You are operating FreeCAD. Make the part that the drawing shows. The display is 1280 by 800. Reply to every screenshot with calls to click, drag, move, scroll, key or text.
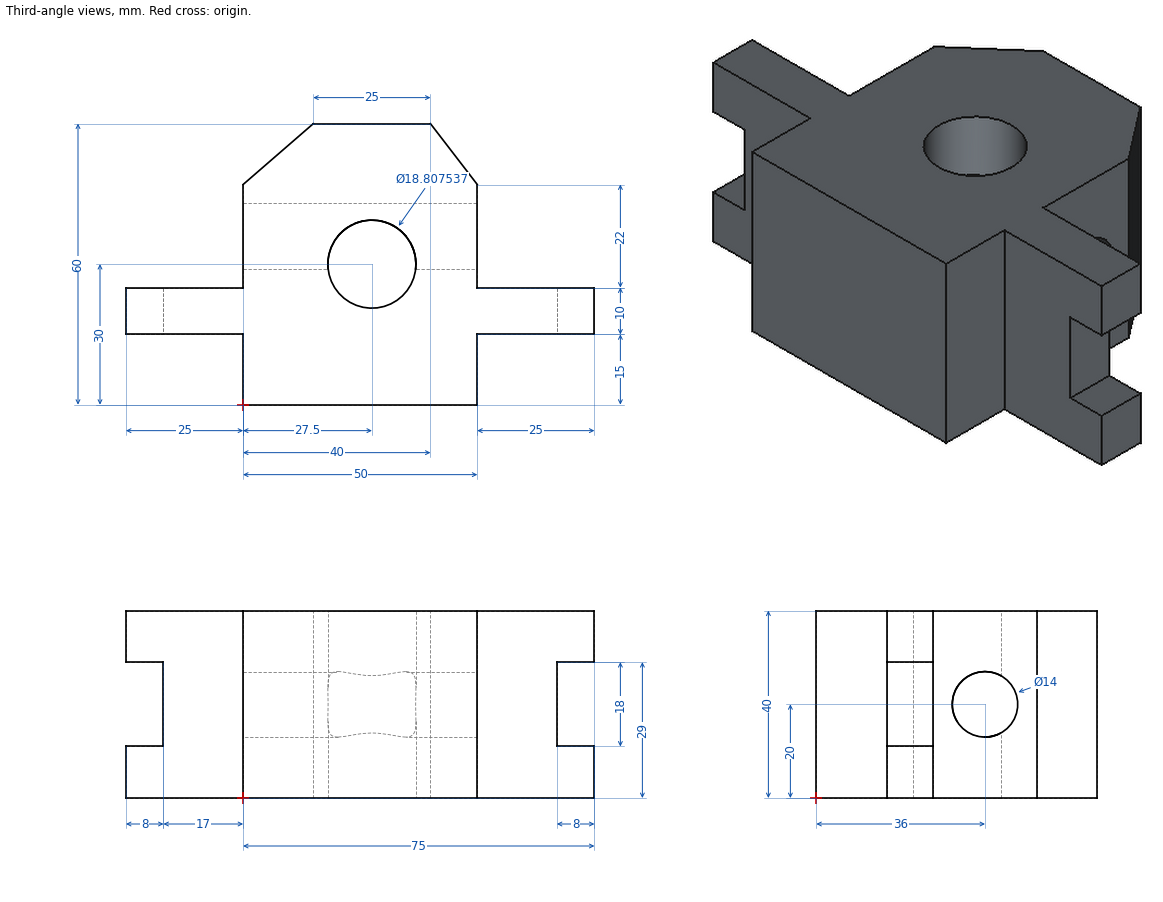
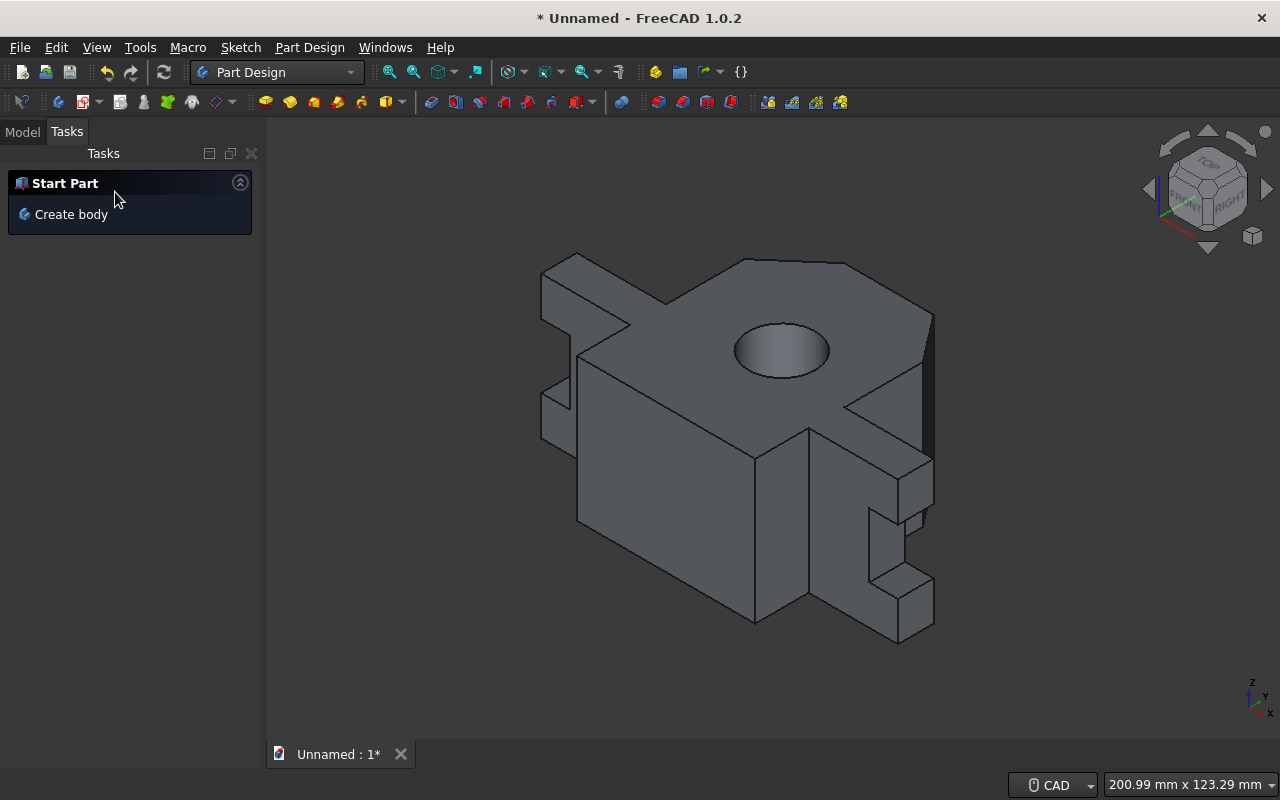
click(895, 413)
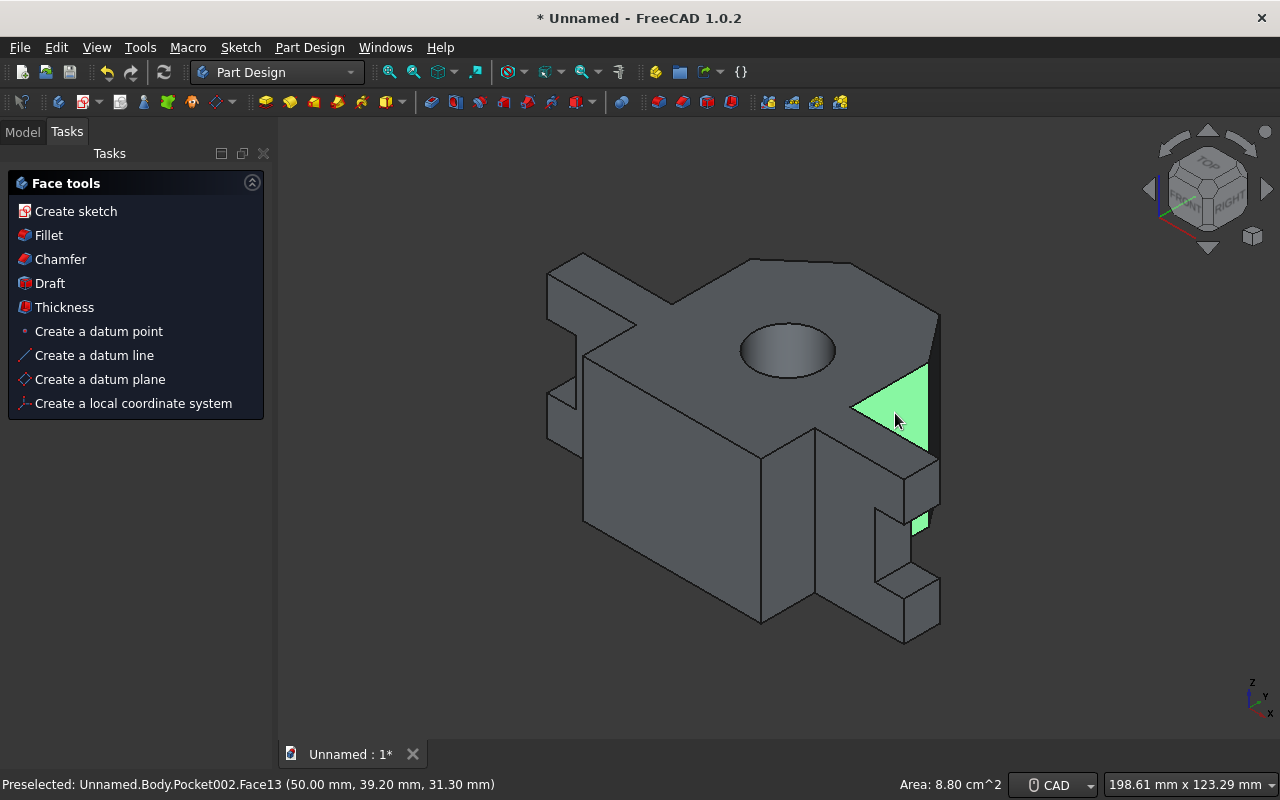
click(84, 102)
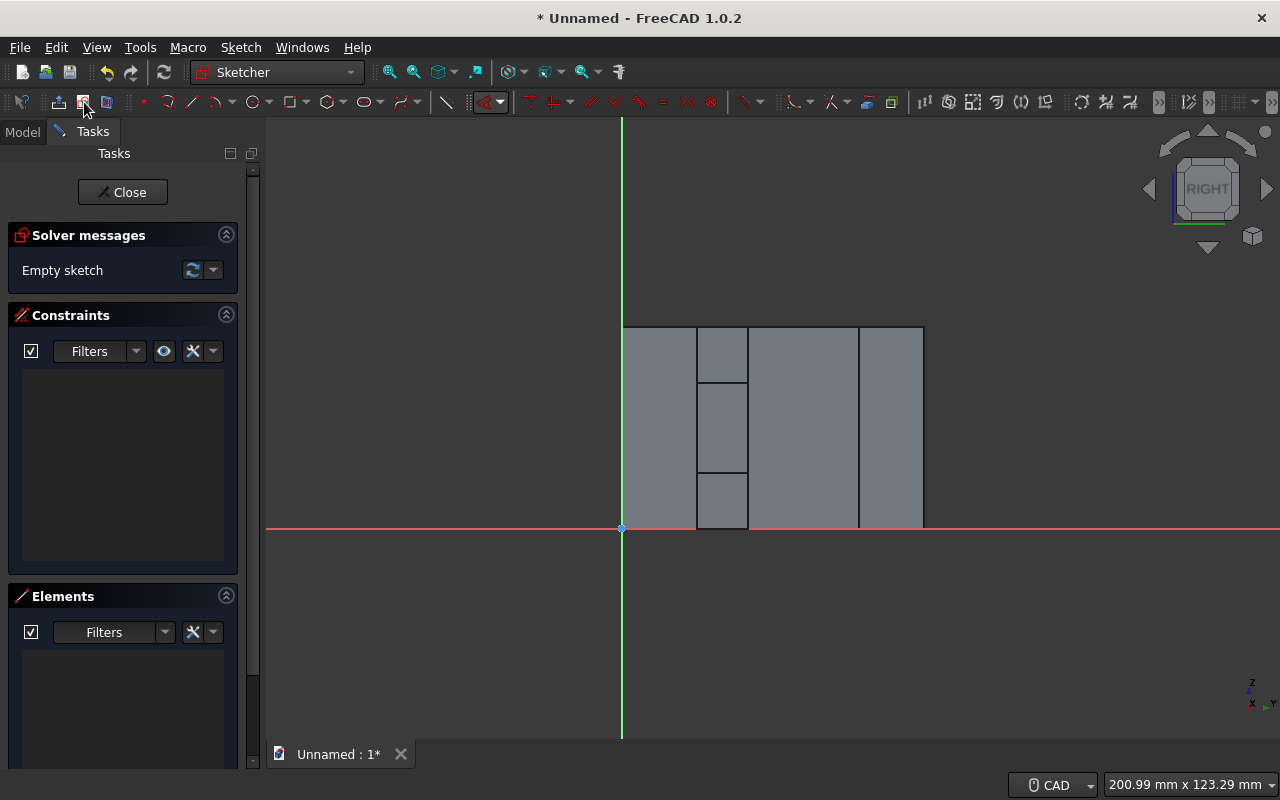
scroll(823, 428, up, 9)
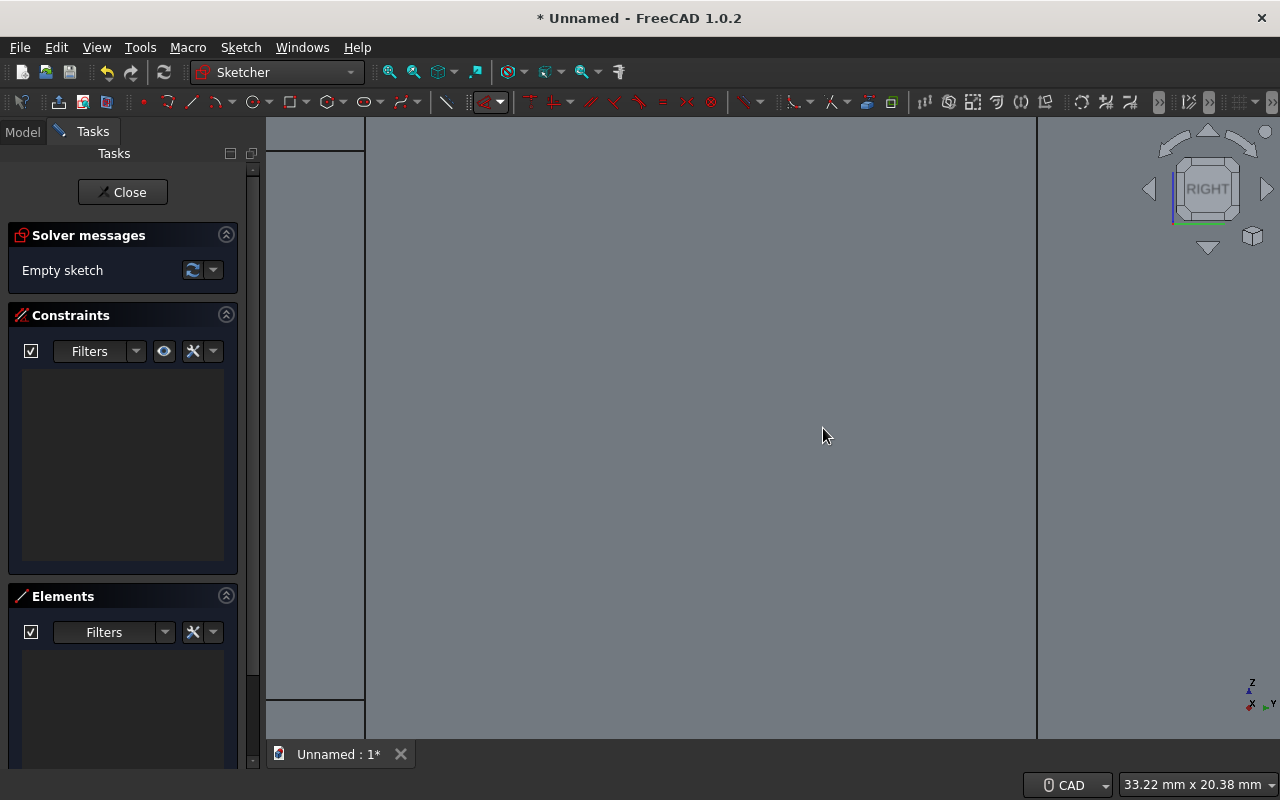
key(g)
key(c)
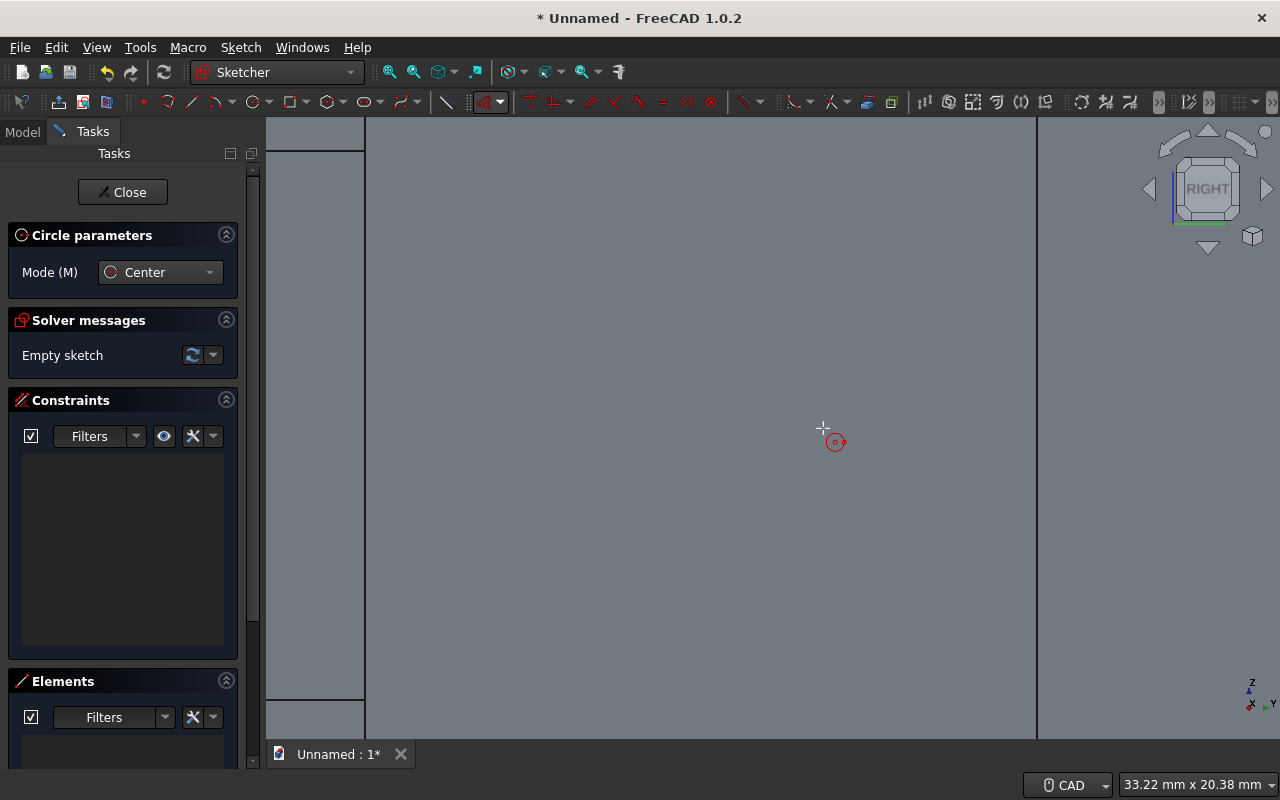
click(701, 425)
move(852, 274)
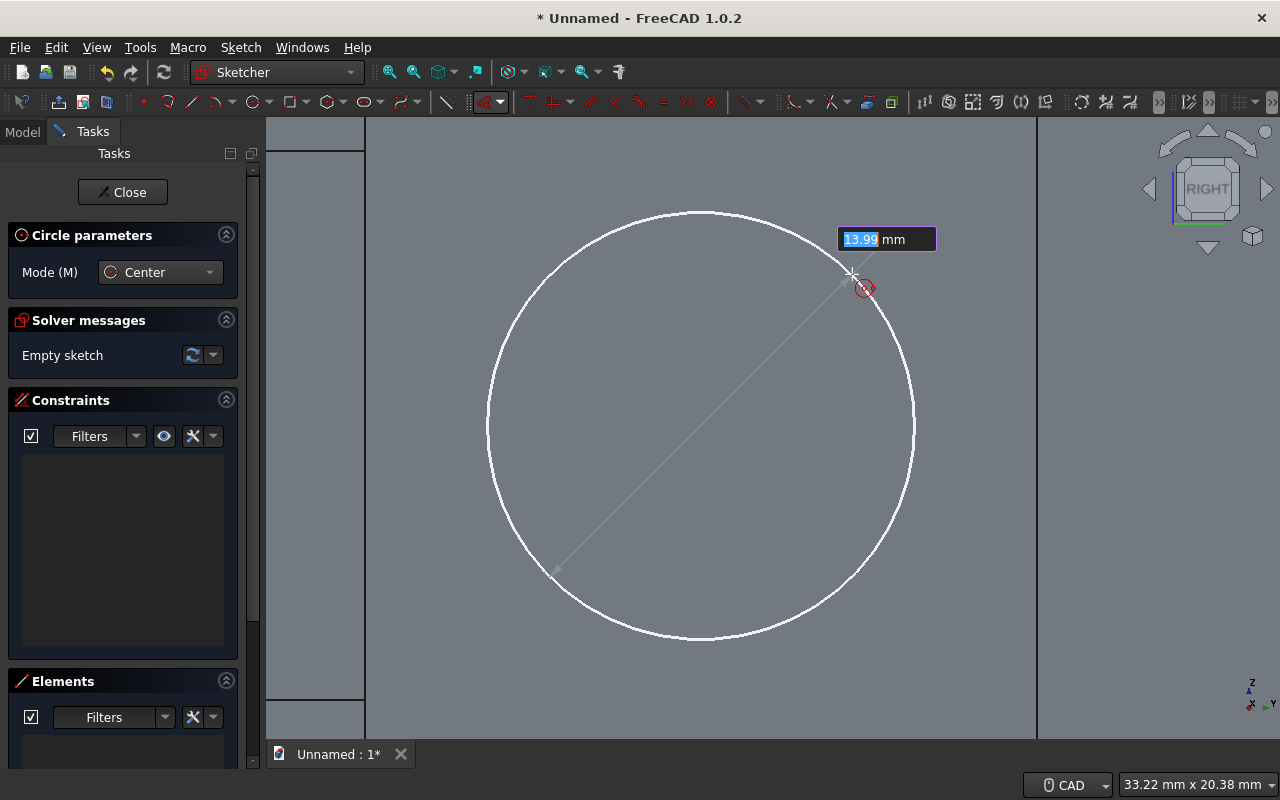
text(14)
key(Return)
key(Escape)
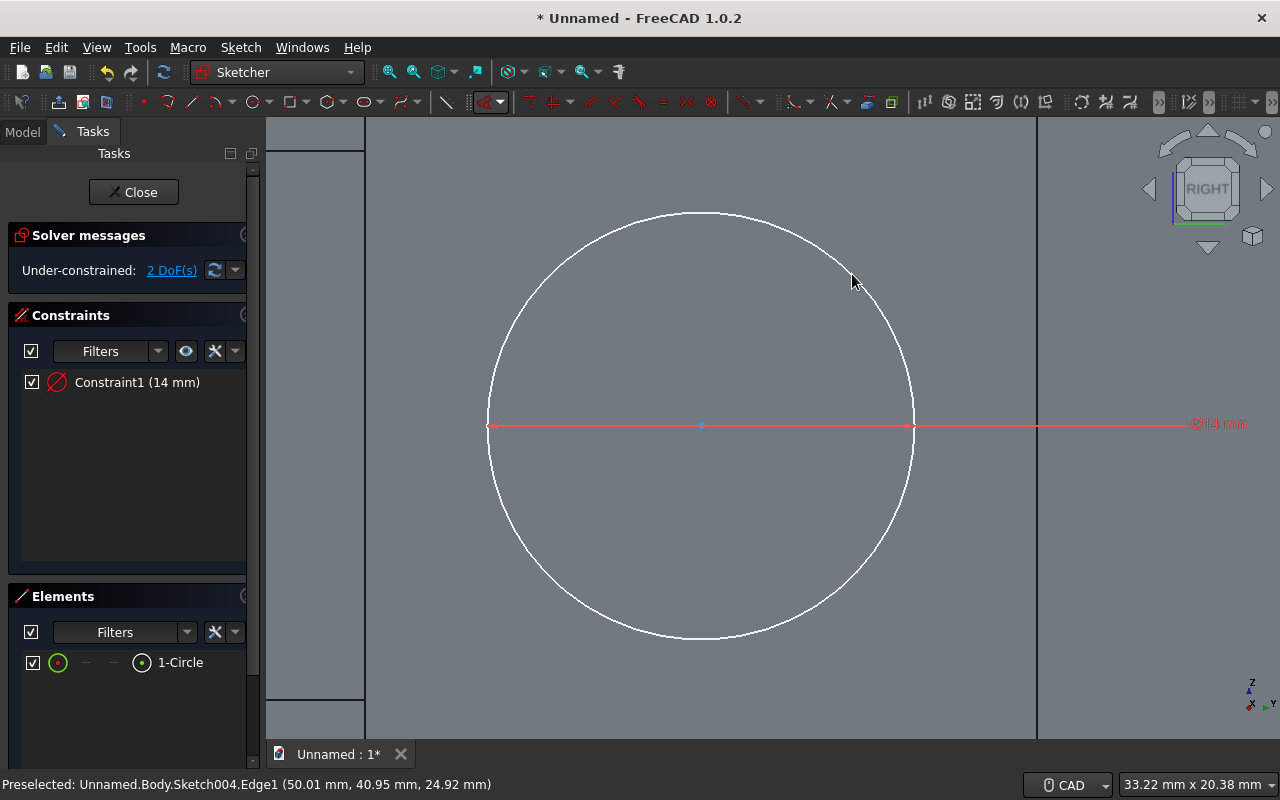
click(701, 426)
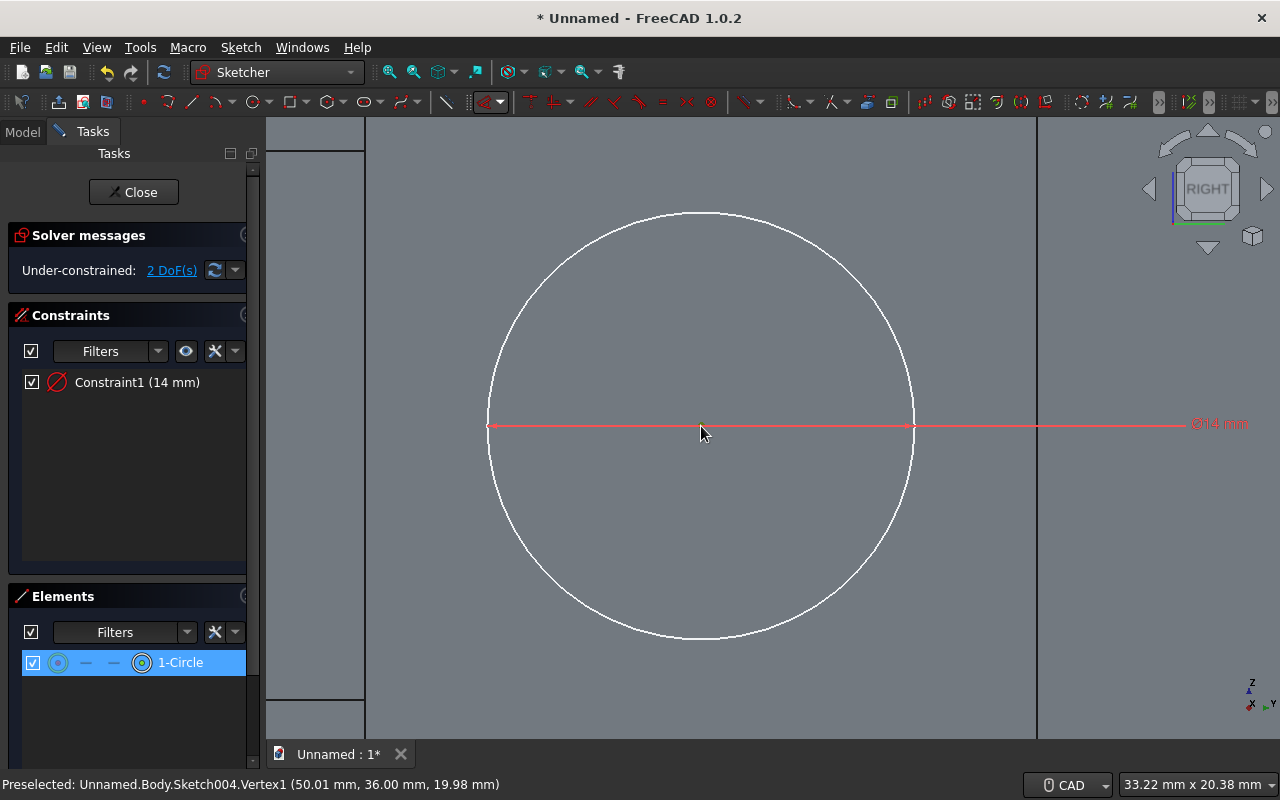
key(l)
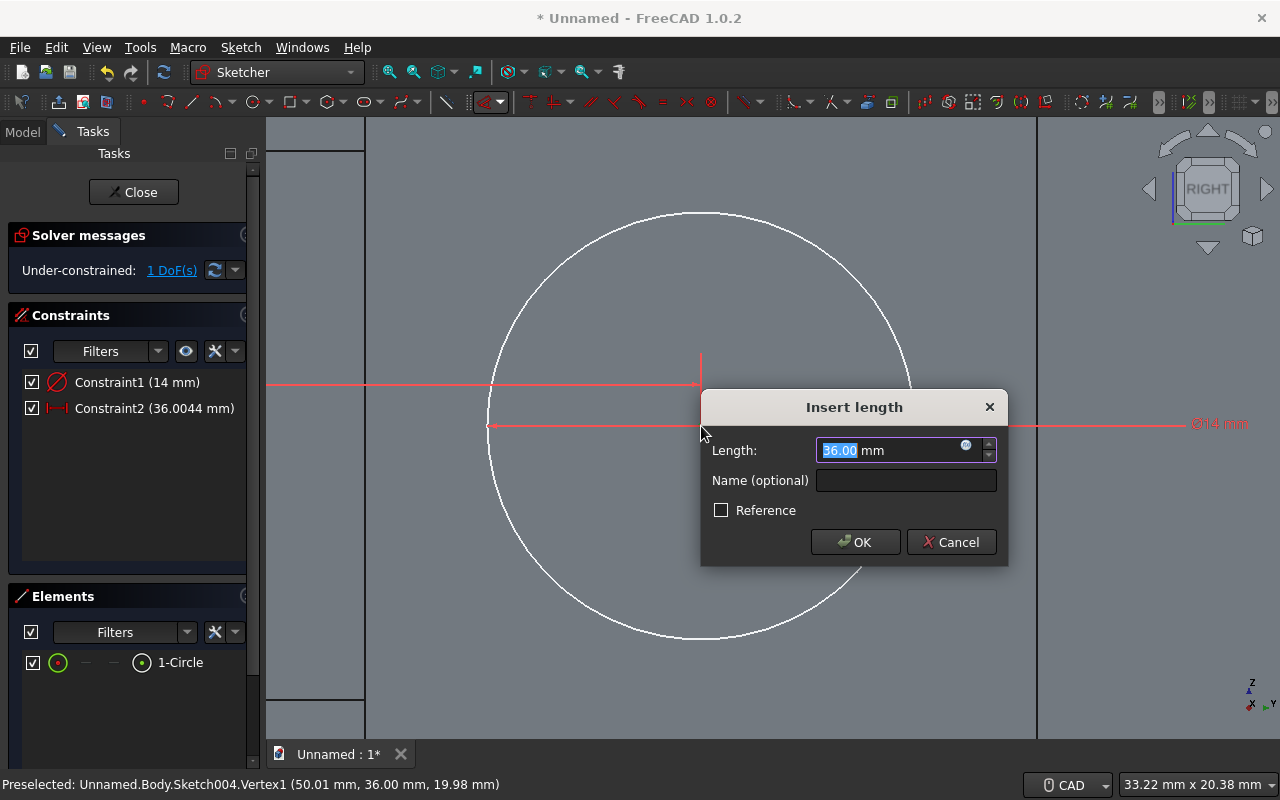
text(36)
key(Return)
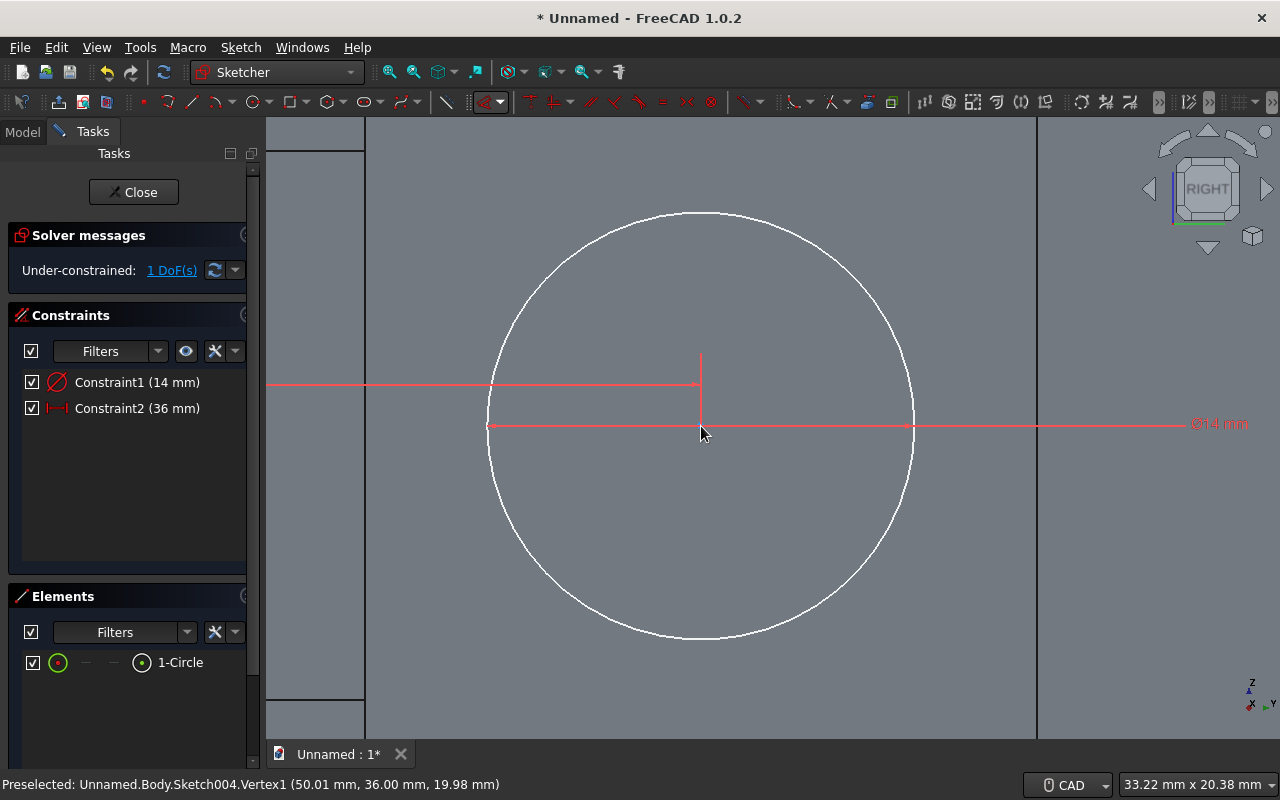
click(701, 426)